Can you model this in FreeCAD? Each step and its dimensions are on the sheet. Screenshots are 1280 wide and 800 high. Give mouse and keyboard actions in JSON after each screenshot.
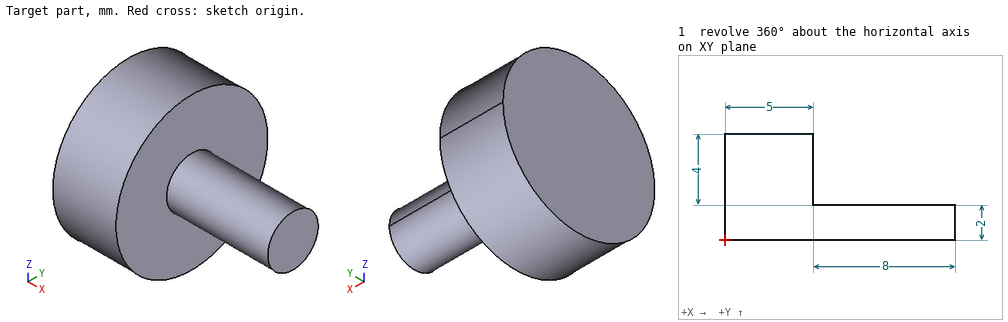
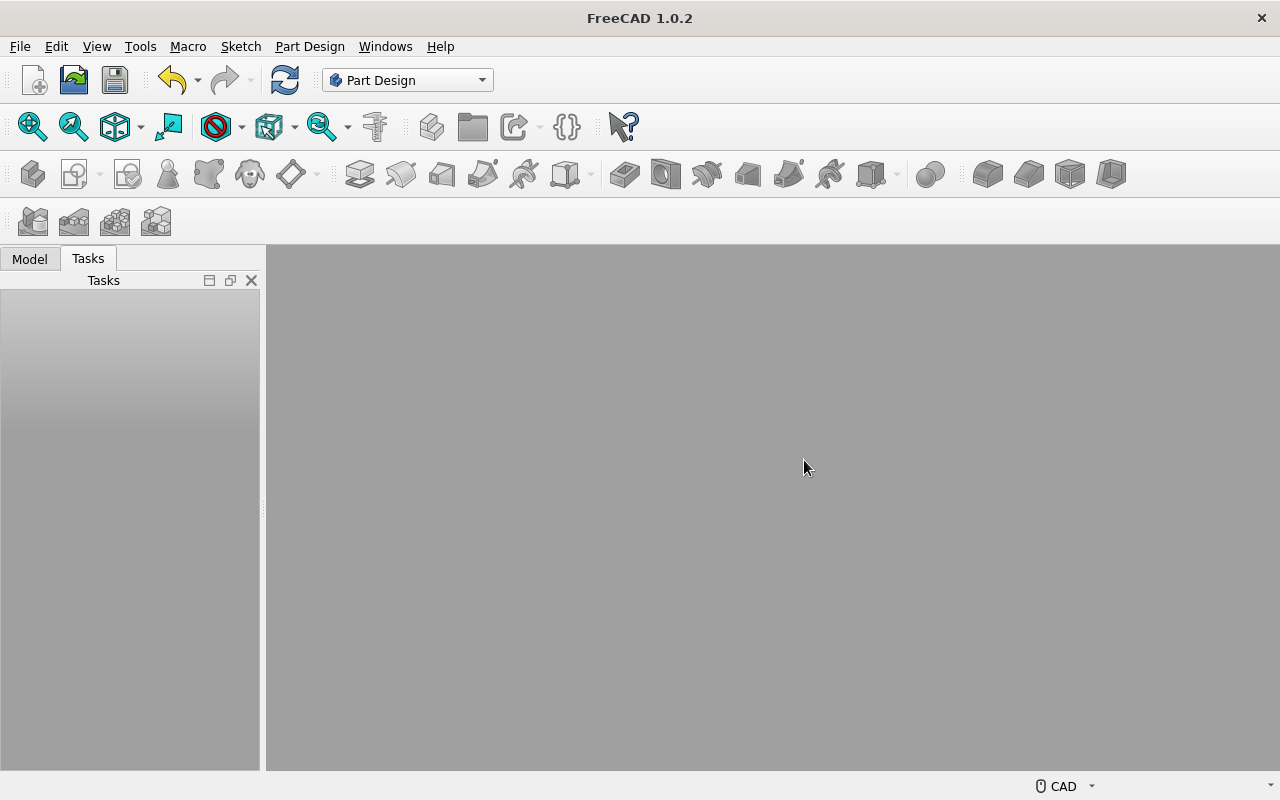
{"action": "key", "text": "ctrl+n"}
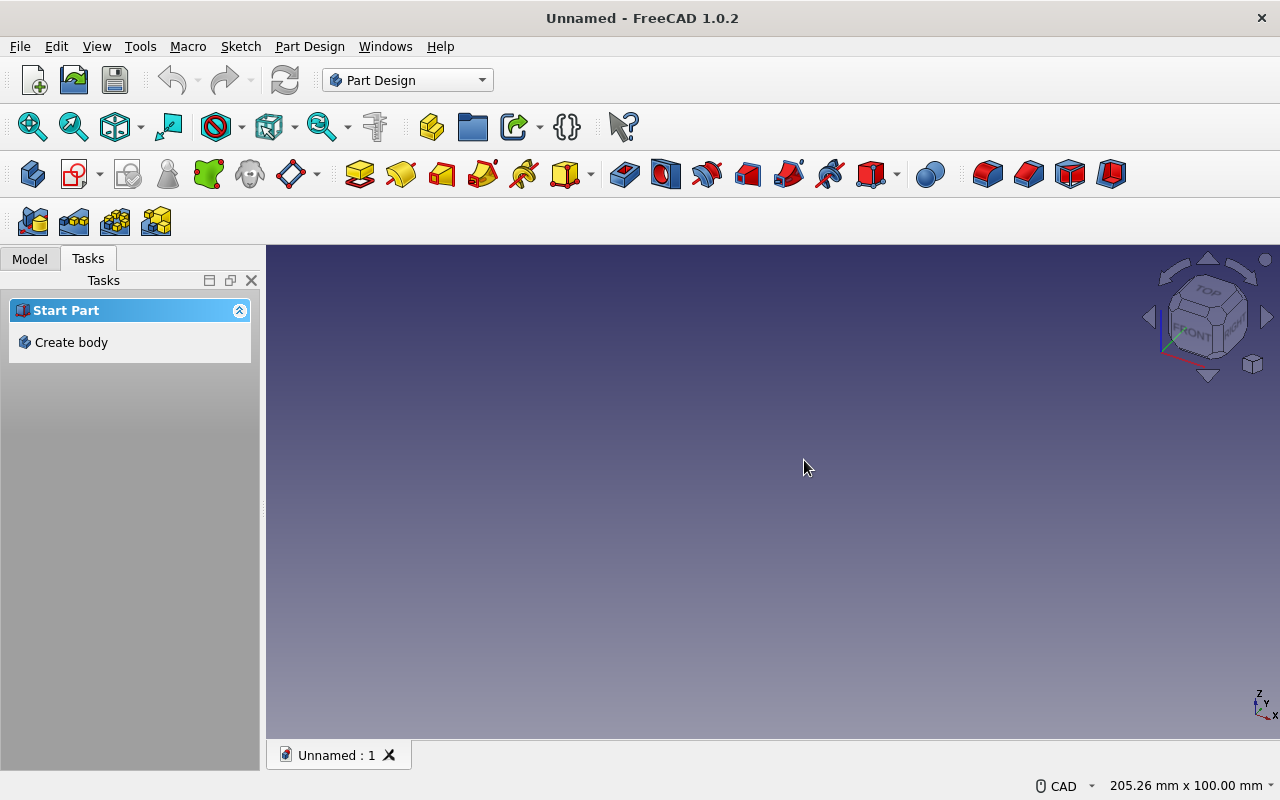
{"action": "left_click", "coordinate": [74, 174]}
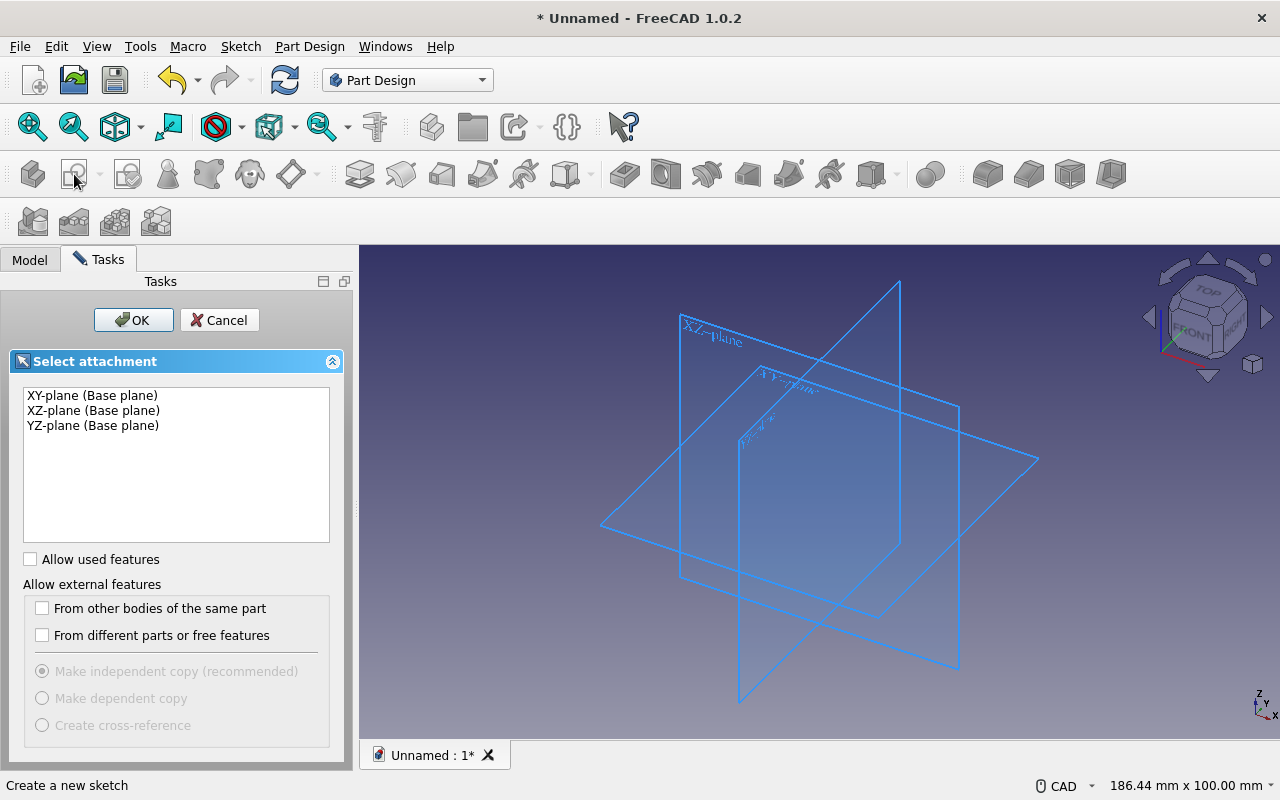
{"action": "left_click", "coordinate": [84, 396]}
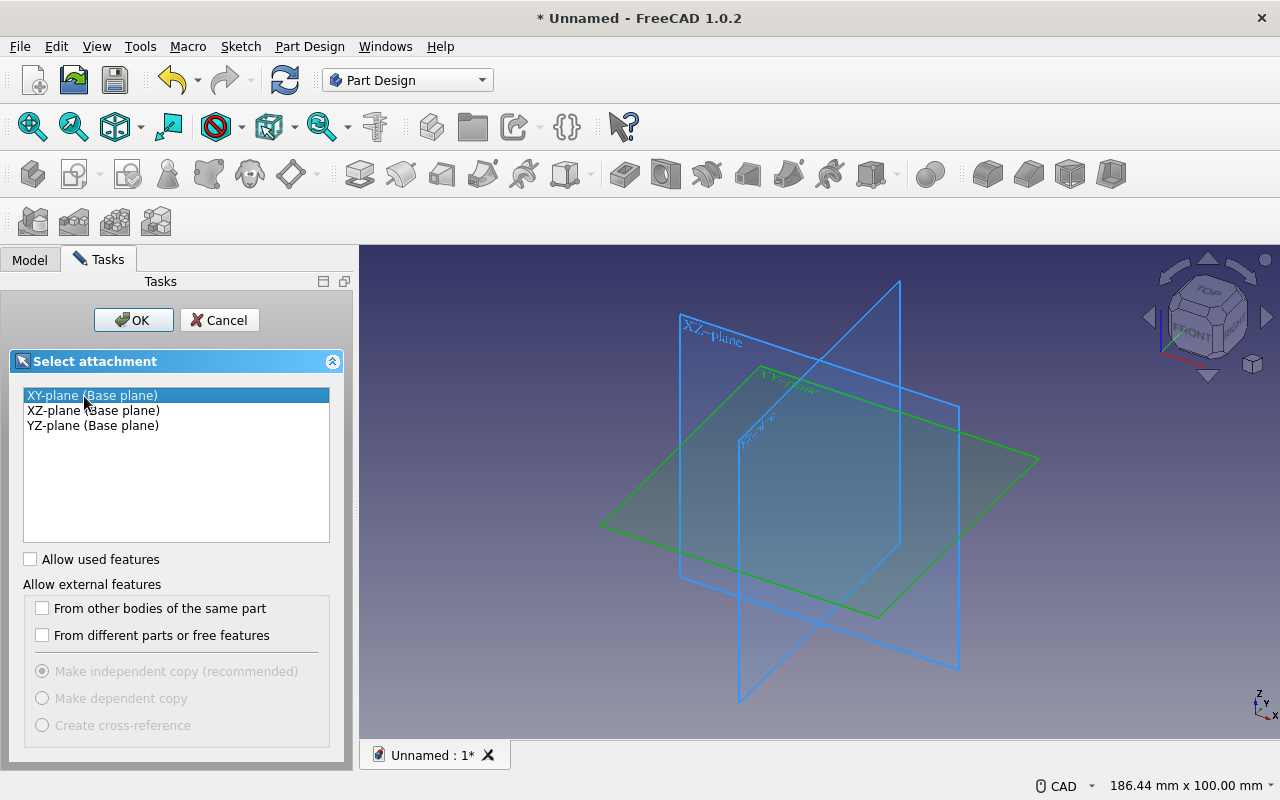
{"action": "left_click", "coordinate": [134, 320]}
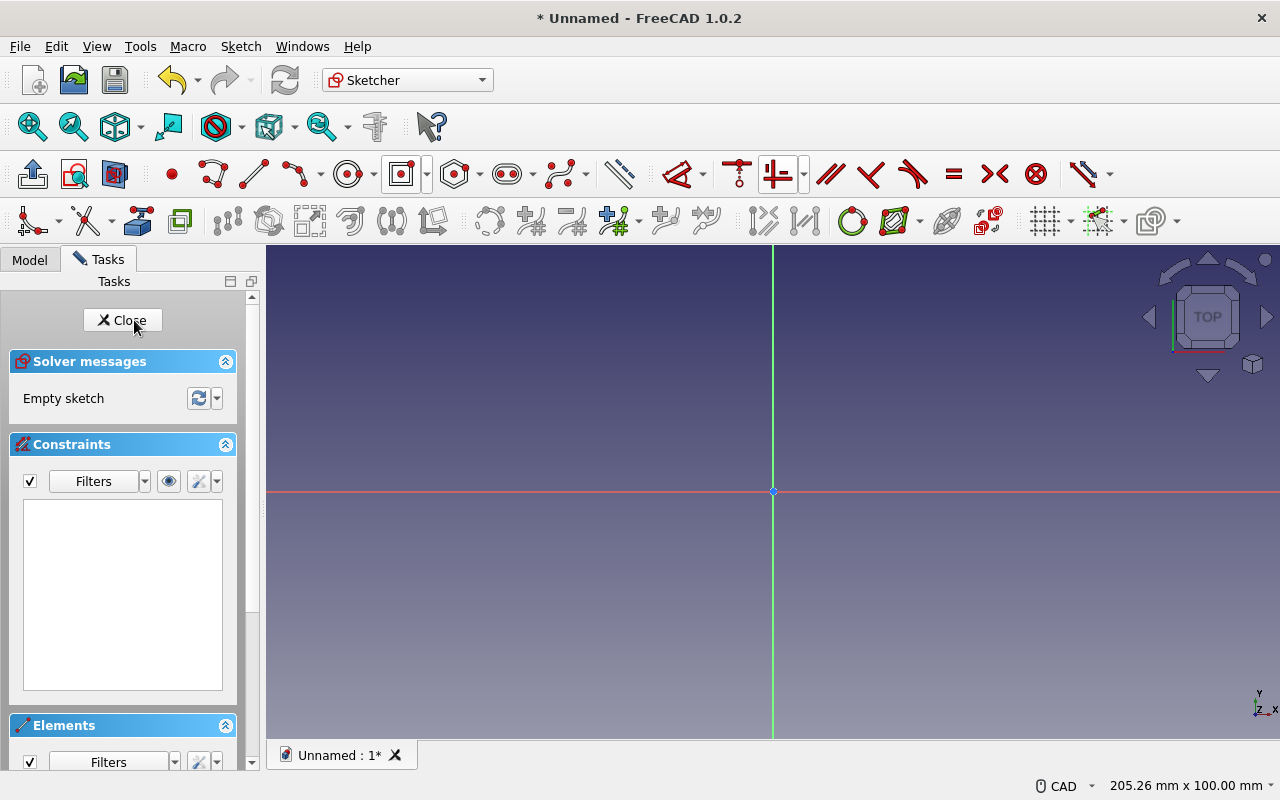
{"action": "scroll", "coordinate": [818, 475], "scroll_direction": "up", "scroll_amount": 11}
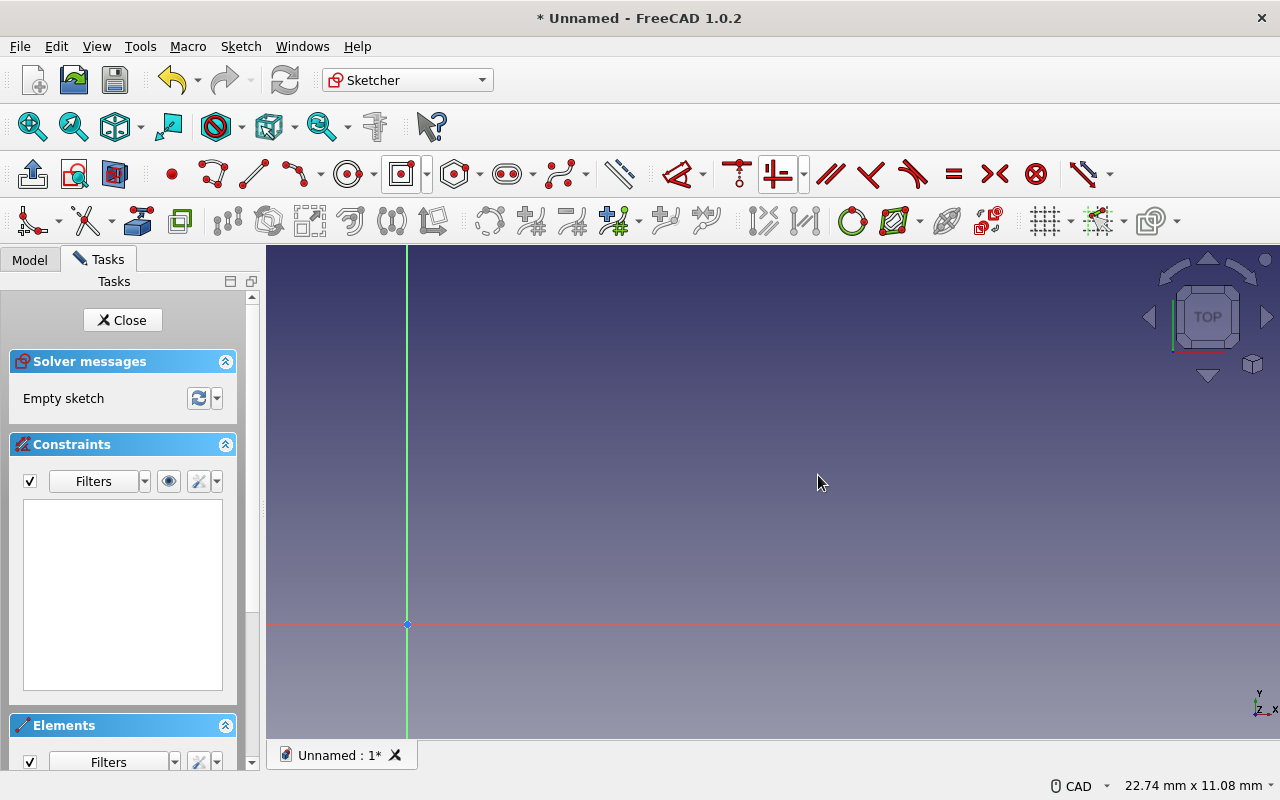
{"action": "key", "text": "g m"}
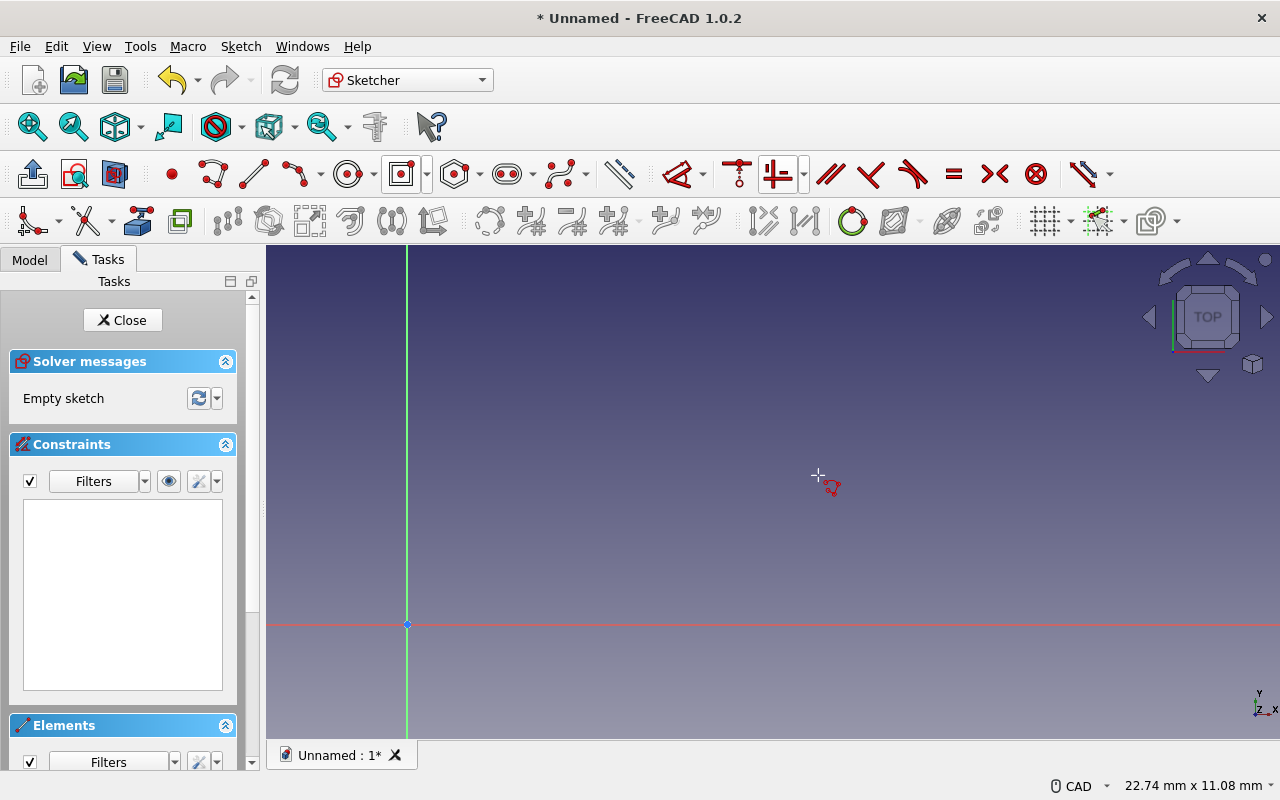
{"action": "left_click", "coordinate": [408, 625]}
{"action": "left_click", "coordinate": [987, 616]}
{"action": "left_click", "coordinate": [987, 536]}
{"action": "left_click", "coordinate": [630, 536]}
{"action": "left_click", "coordinate": [630, 357]}
{"action": "left_click", "coordinate": [417, 357]}
{"action": "left_click", "coordinate": [408, 625]}
{"action": "key", "text": "Escape"}
{"action": "key", "text": "Escape"}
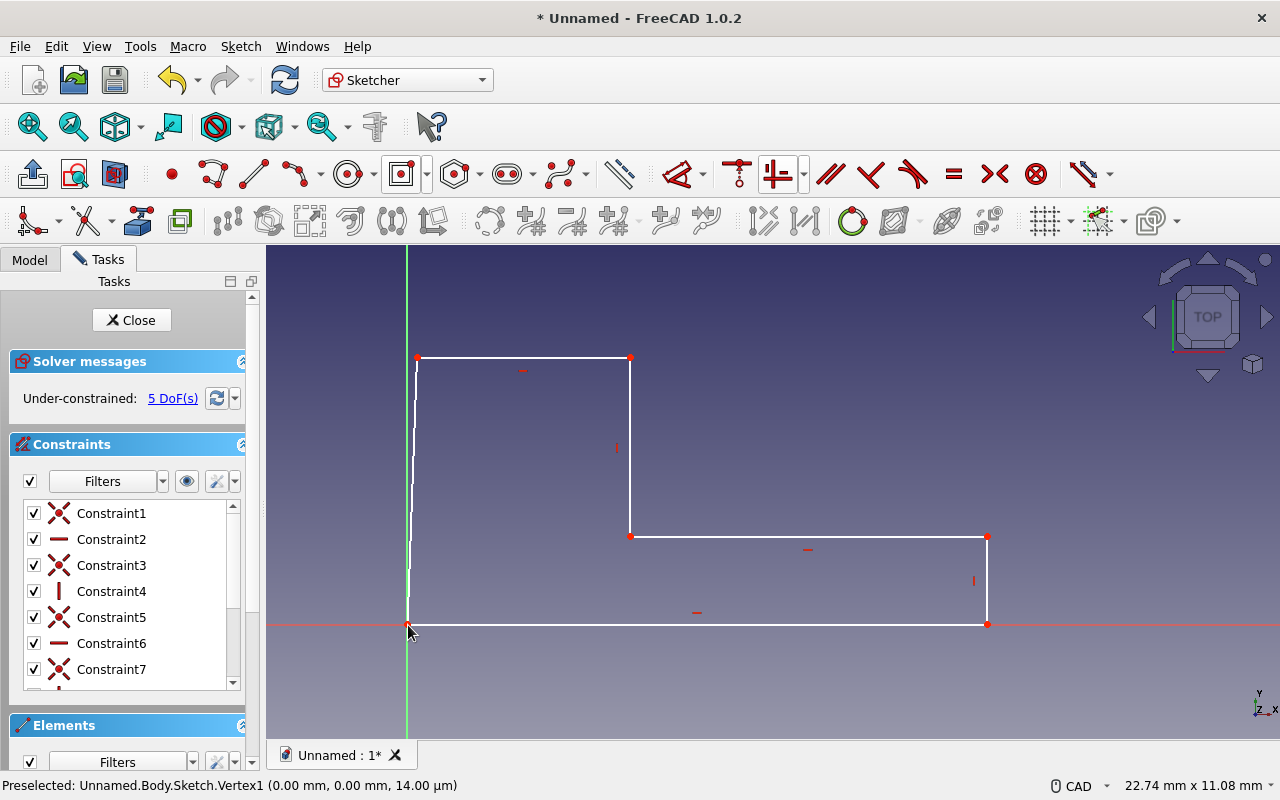
{"action": "left_click", "coordinate": [410, 545]}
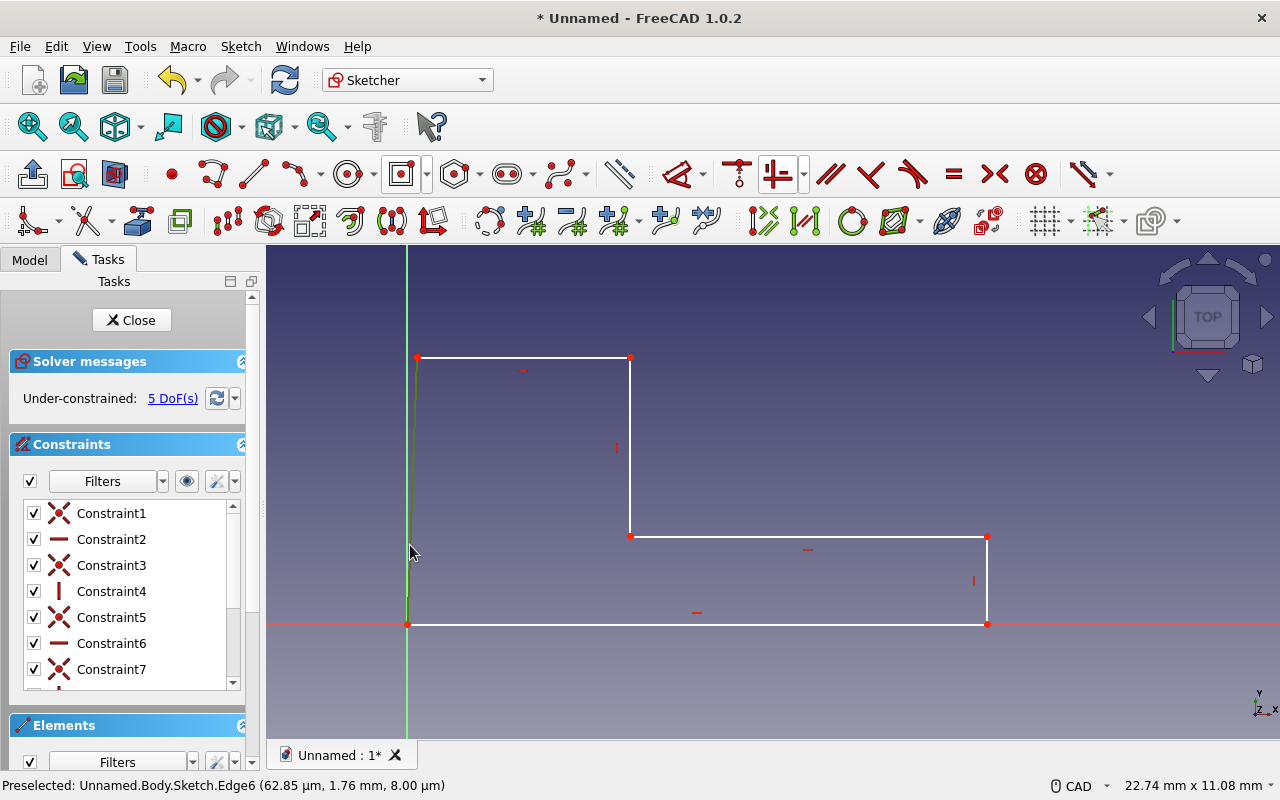
{"action": "key", "text": "v"}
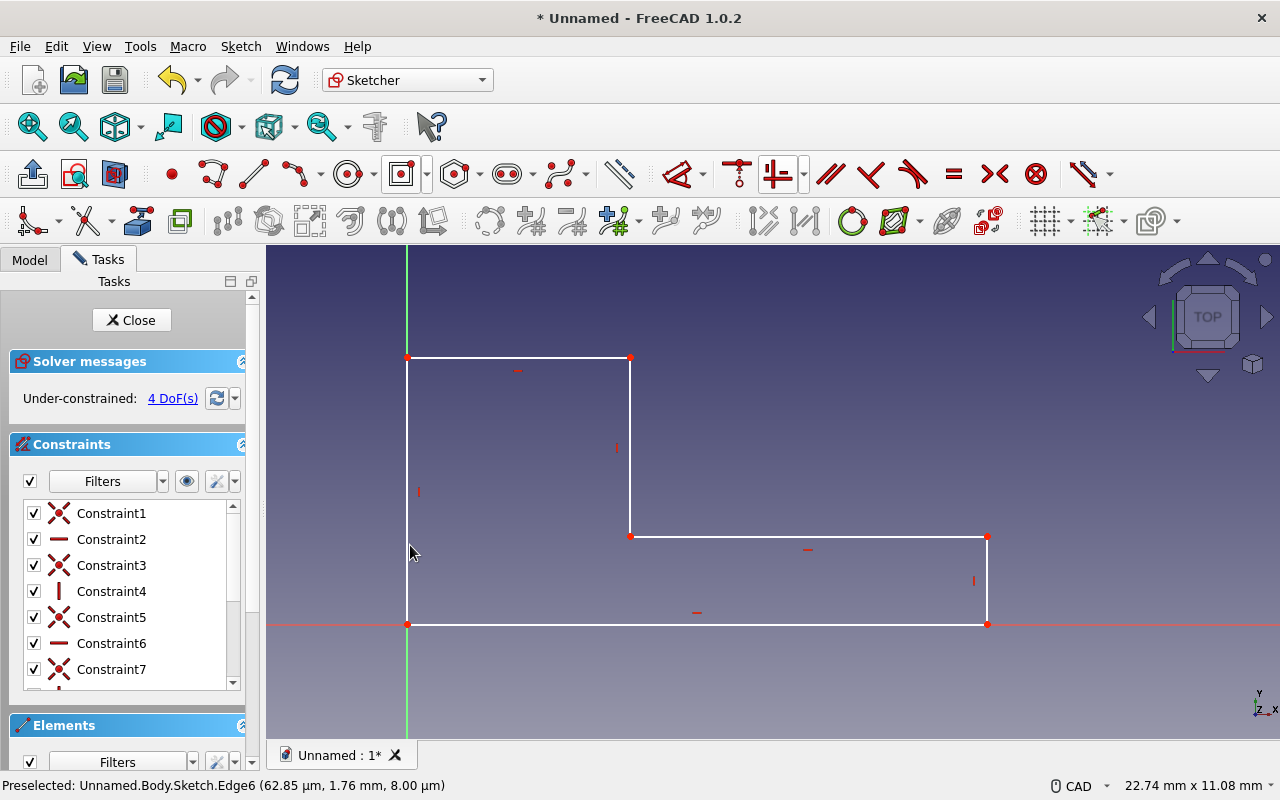
{"action": "left_click", "coordinate": [987, 598]}